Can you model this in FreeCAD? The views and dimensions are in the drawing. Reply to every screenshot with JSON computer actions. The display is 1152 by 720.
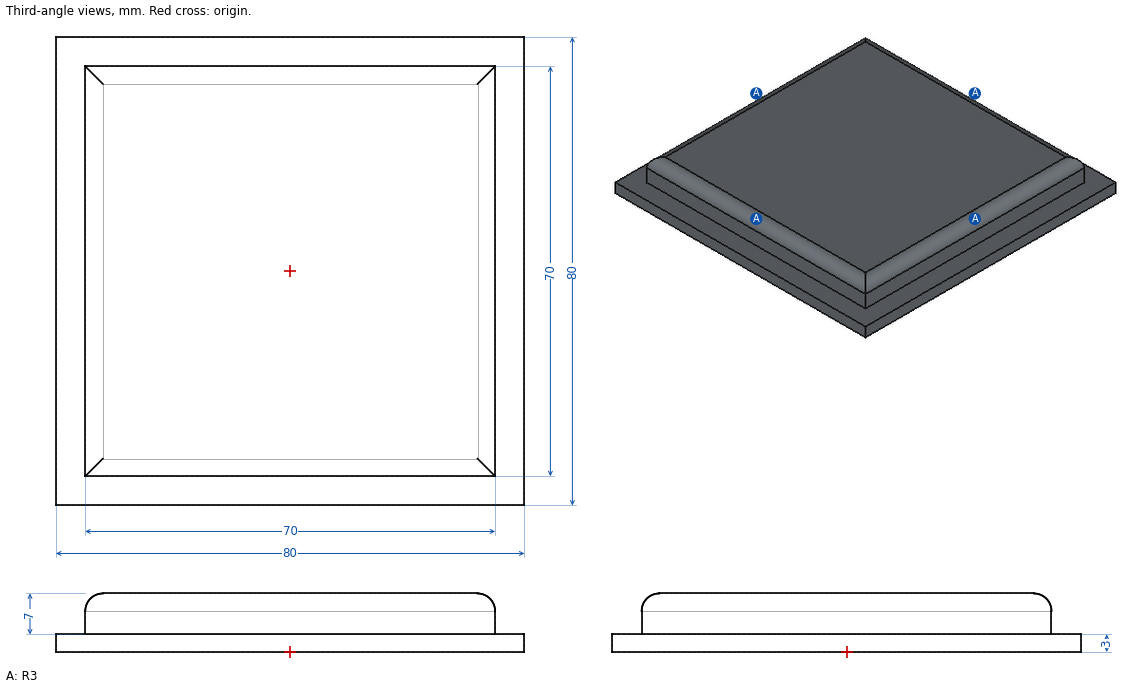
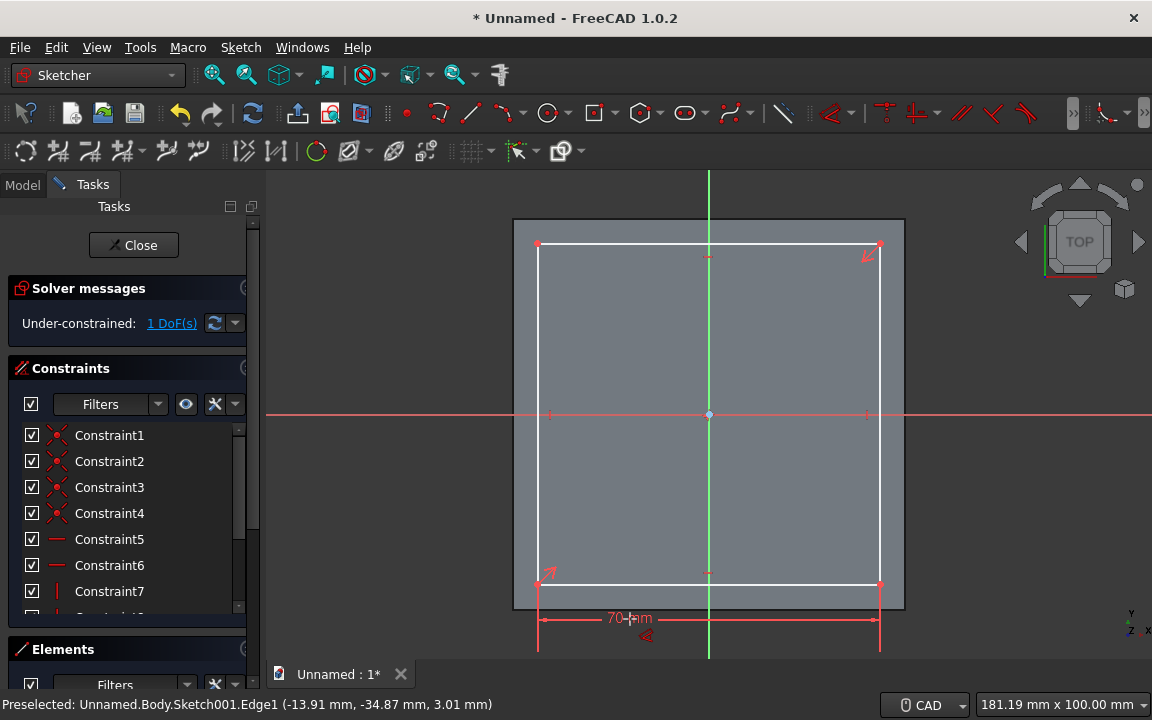
{"action": "left_click", "coordinate": [880, 483]}
{"action": "left_click", "coordinate": [914, 336]}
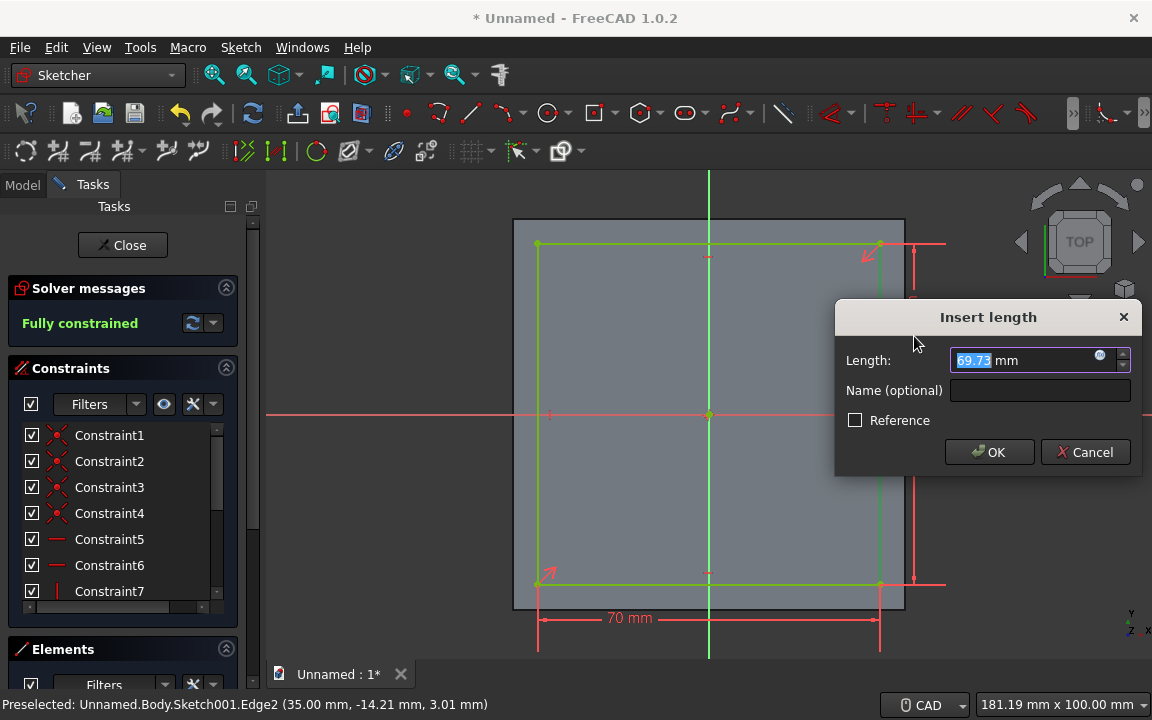
{"action": "type", "text": "70"}
{"action": "key", "text": "Return"}
{"action": "key", "text": "Escape"}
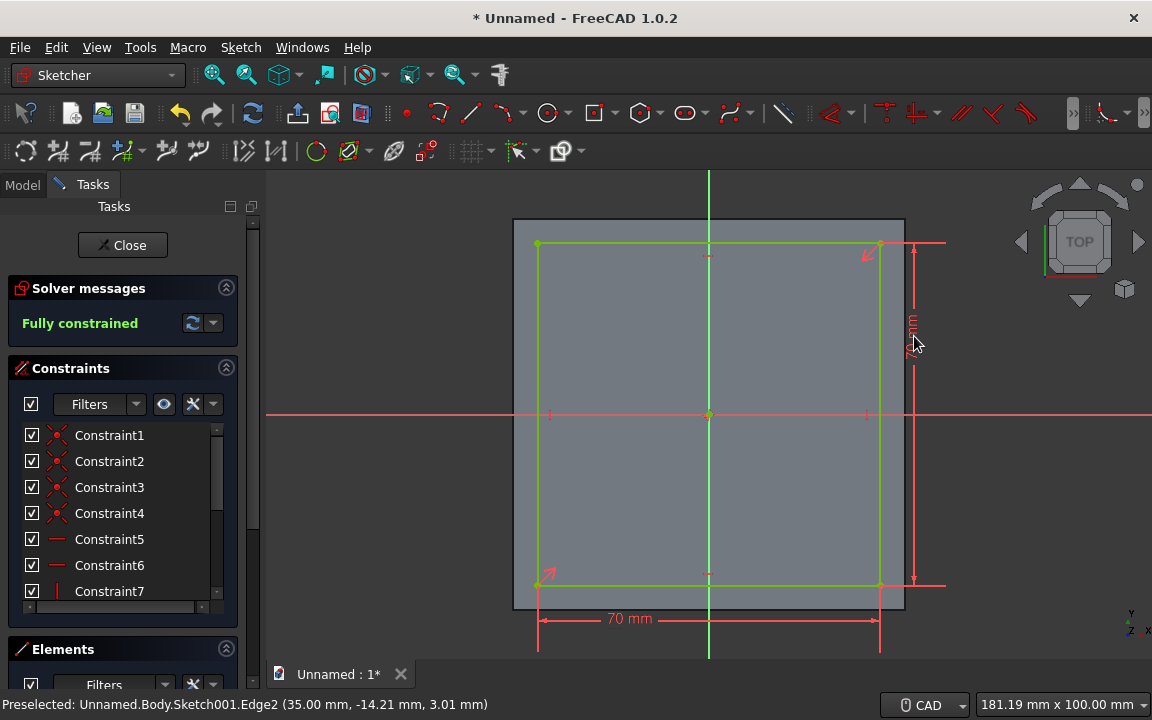
{"action": "left_click", "coordinate": [123, 245]}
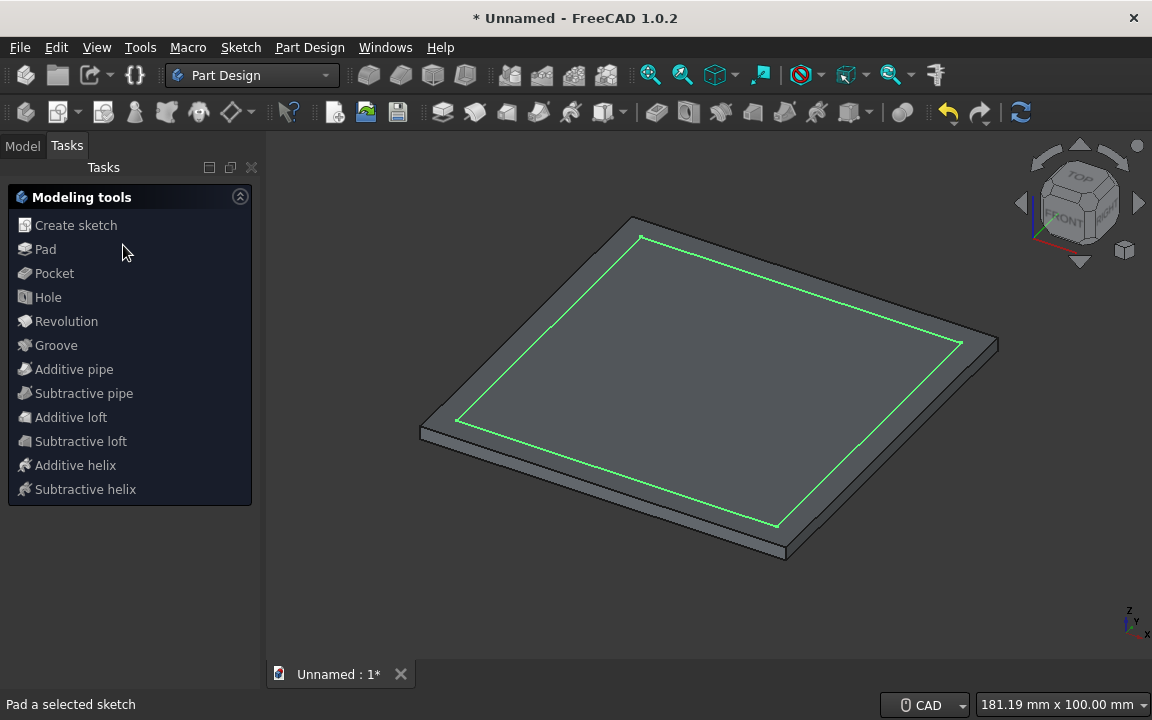
{"action": "left_click", "coordinate": [444, 112]}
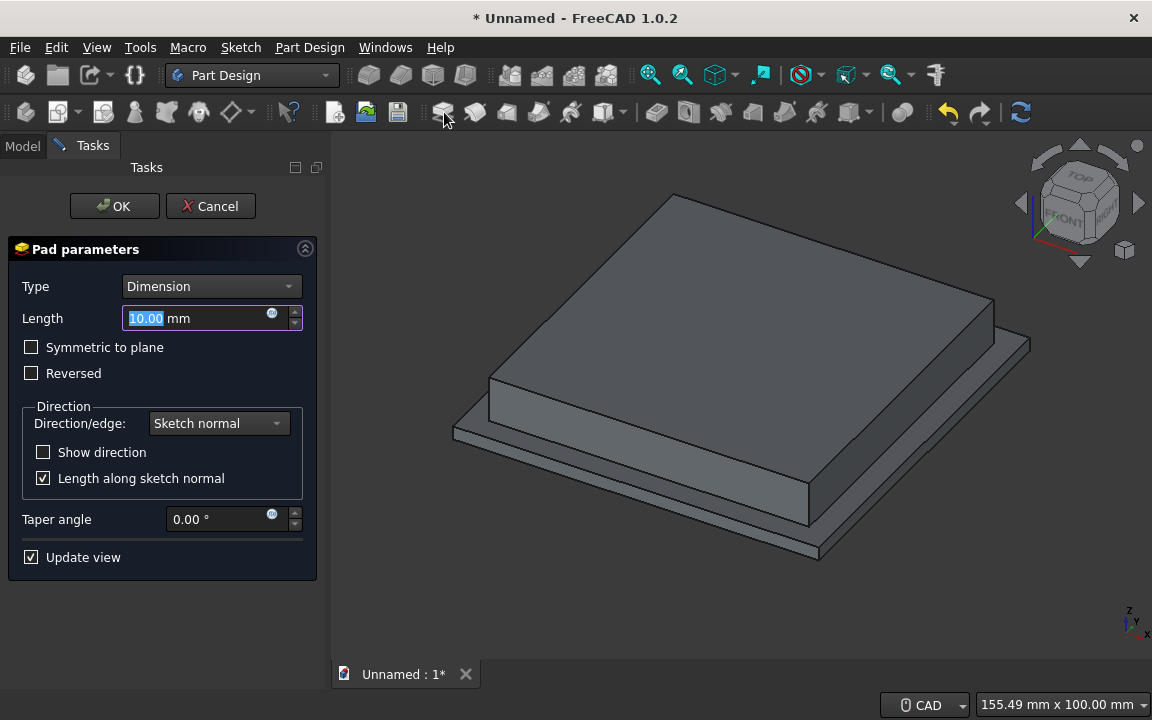
{"action": "type", "text": "7"}
{"action": "key", "text": "Tab"}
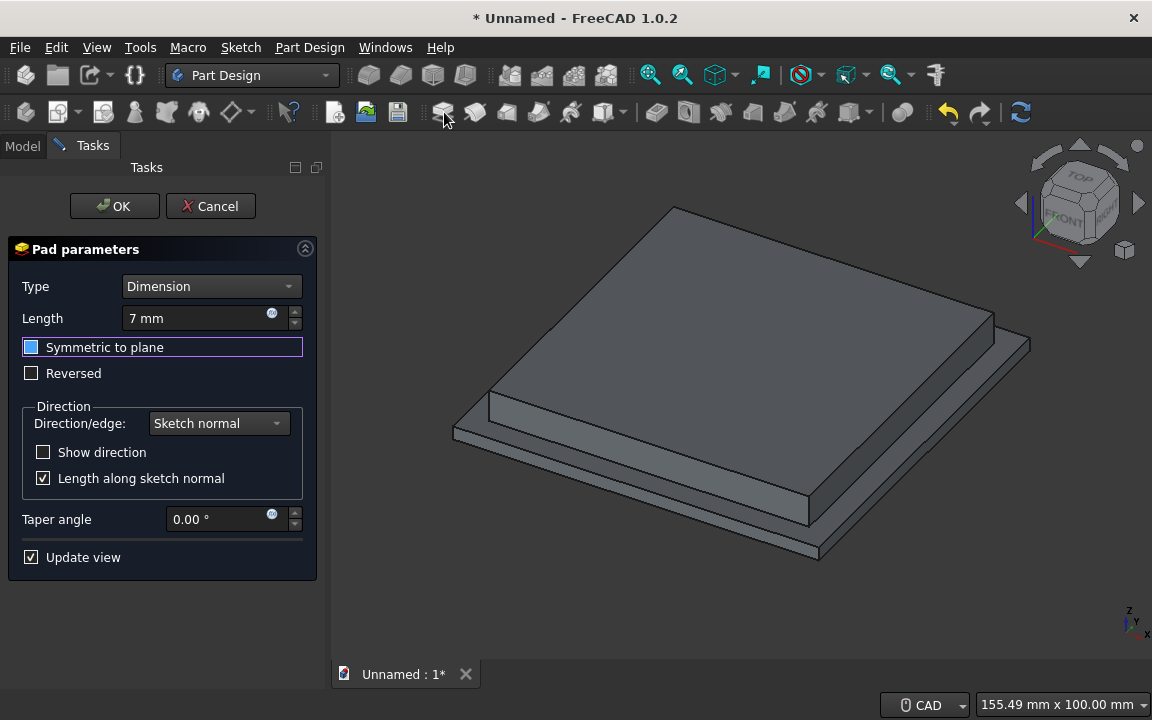
{"action": "left_click", "coordinate": [115, 206]}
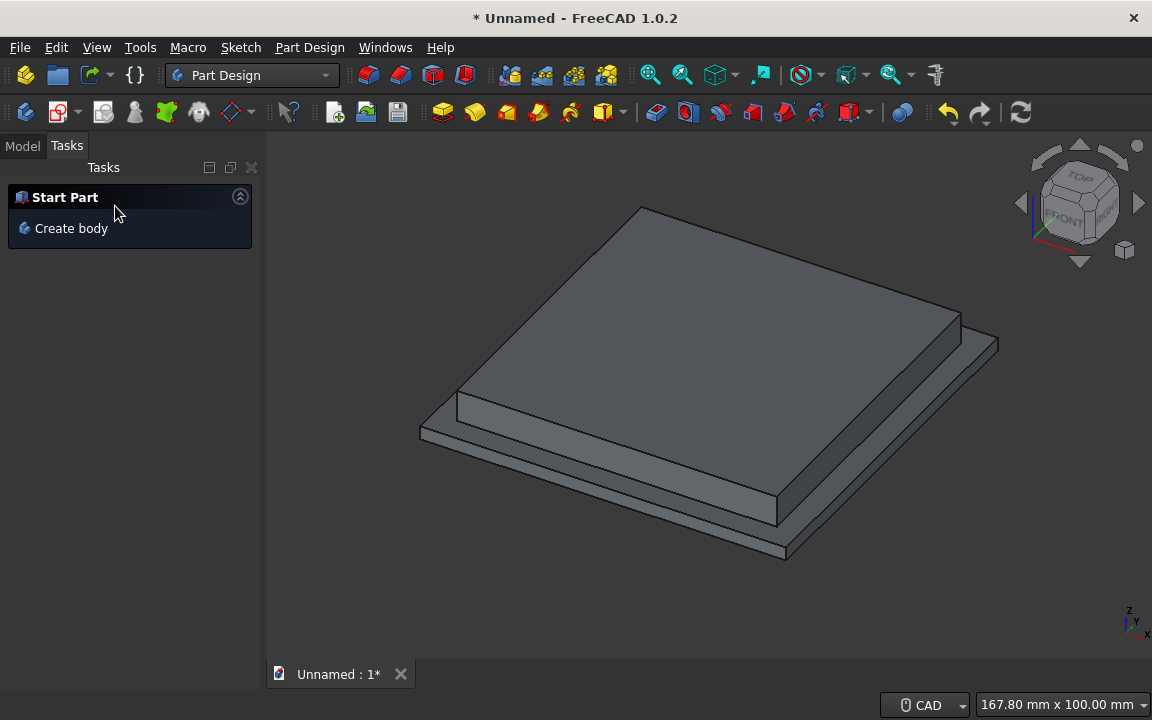
{"action": "left_click", "coordinate": [709, 351]}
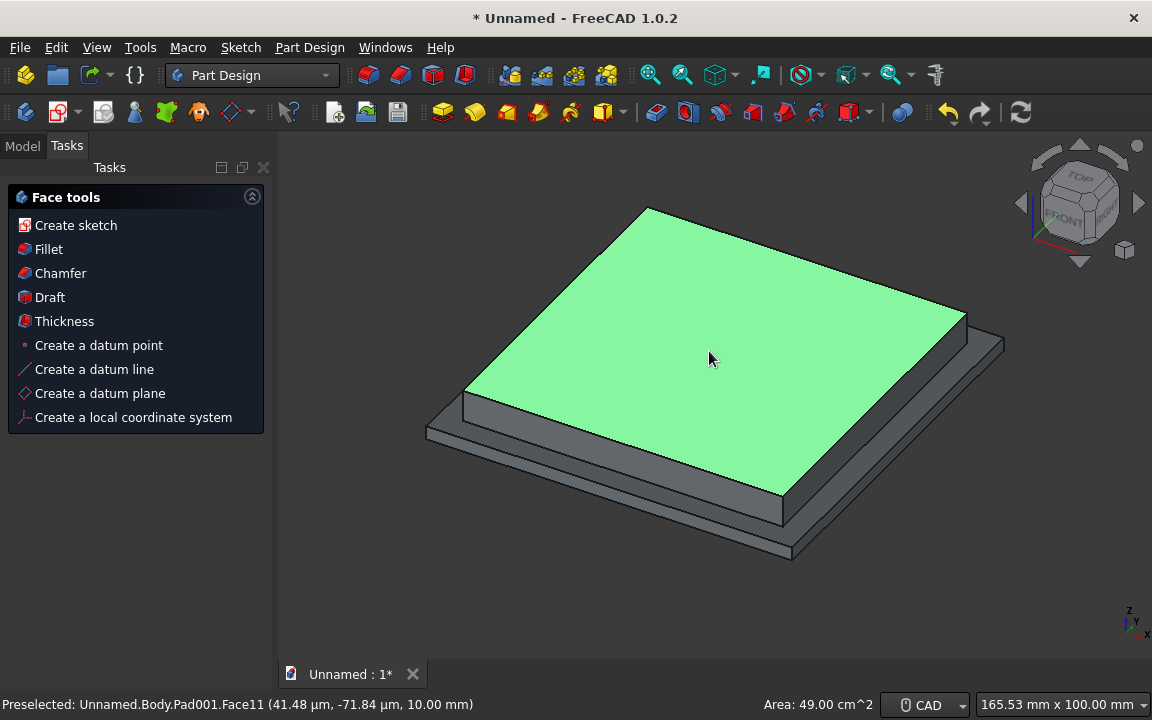
{"action": "left_click", "coordinate": [370, 76]}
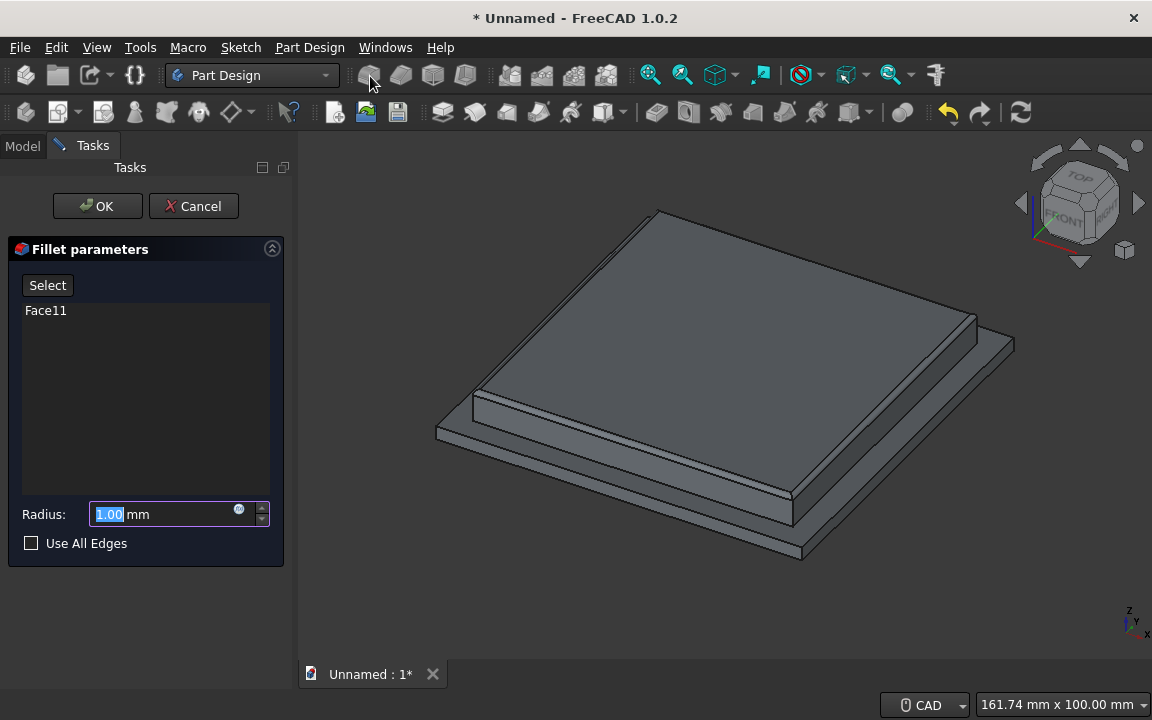
{"action": "type", "text": "3"}
{"action": "key", "text": "Tab"}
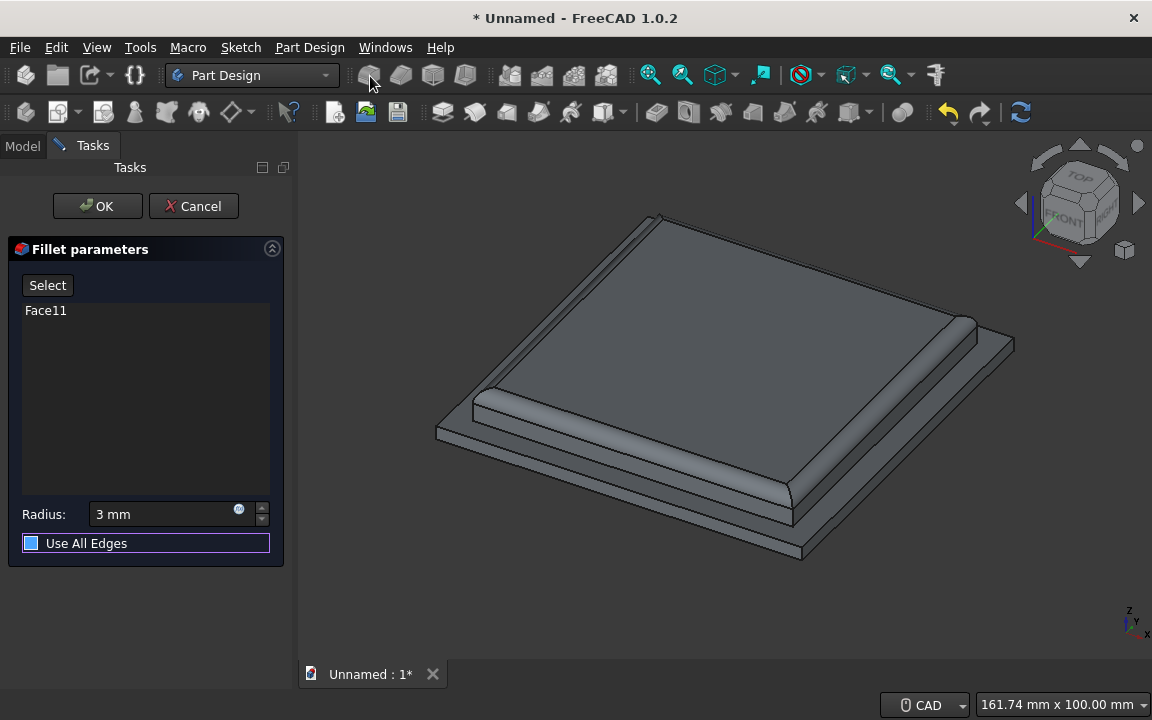
{"action": "left_click", "coordinate": [98, 206]}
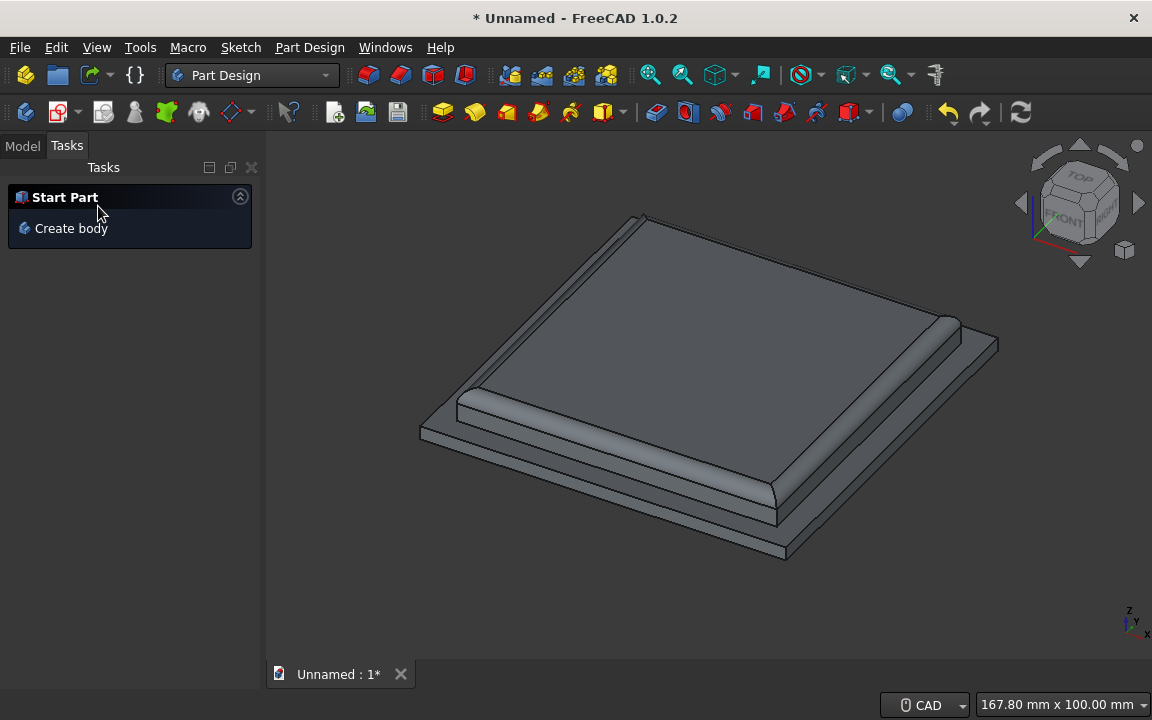
{"action": "key", "text": "0"}